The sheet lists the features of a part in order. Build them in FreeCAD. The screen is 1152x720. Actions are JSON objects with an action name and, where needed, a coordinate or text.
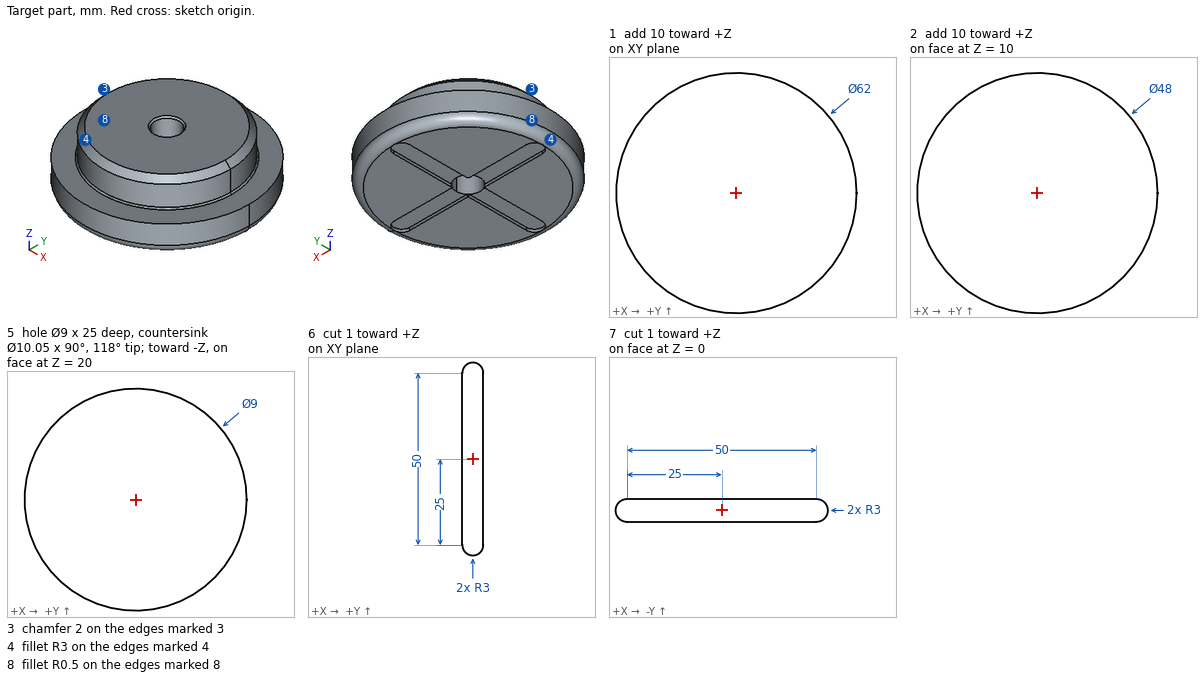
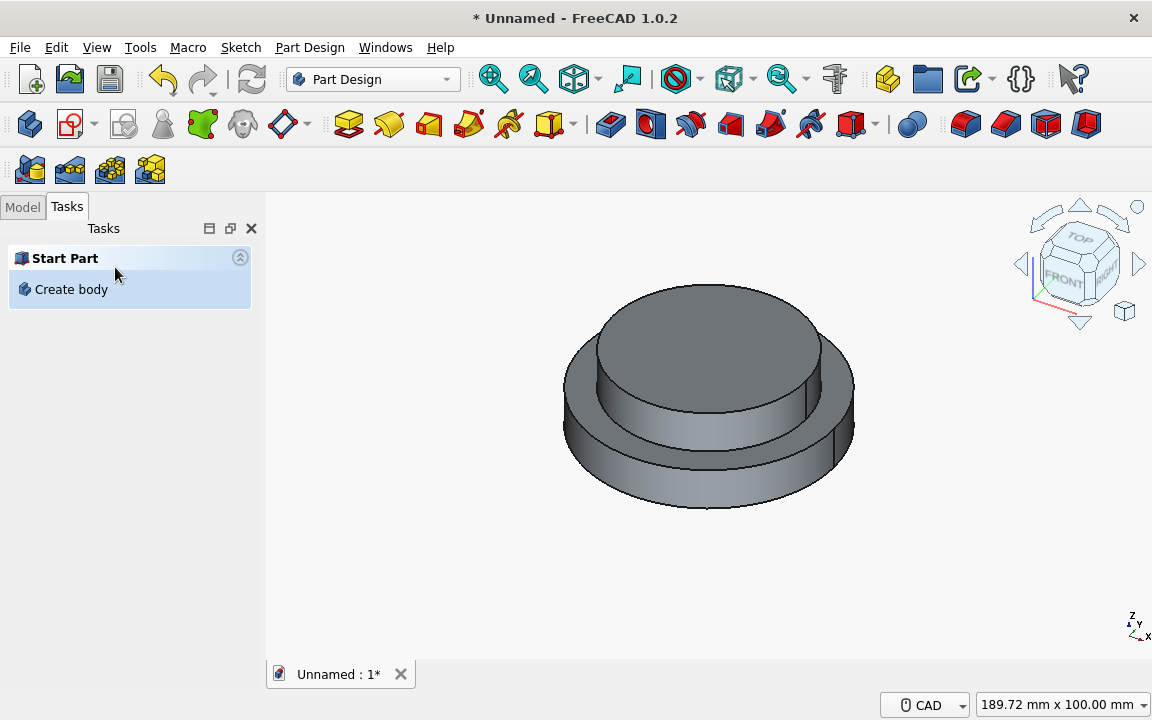
{"action": "left_click", "coordinate": [598, 355]}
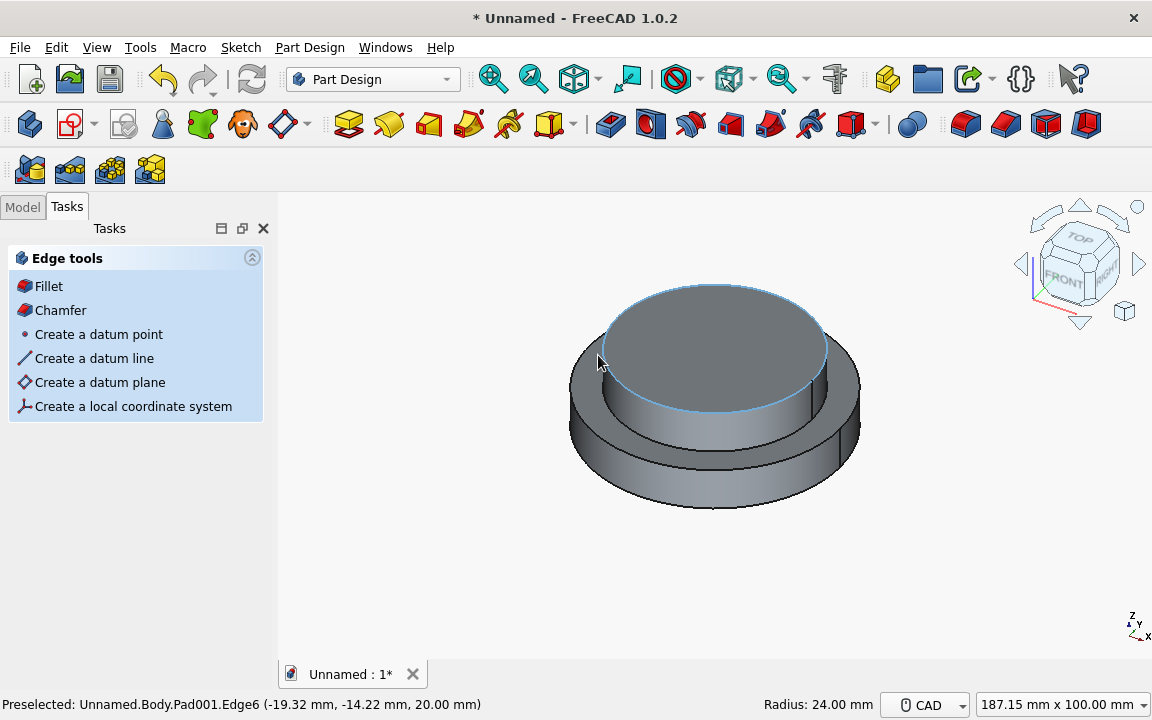
{"action": "left_click", "coordinate": [1006, 124]}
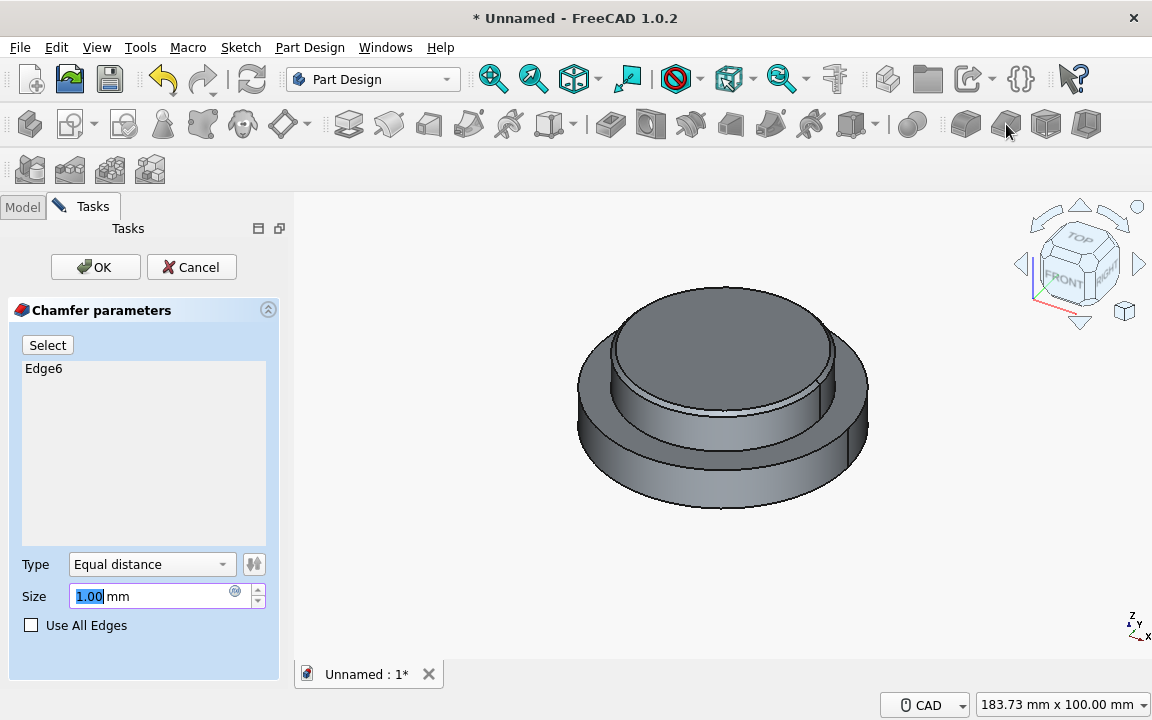
{"action": "type", "text": "2"}
{"action": "key", "text": "Tab"}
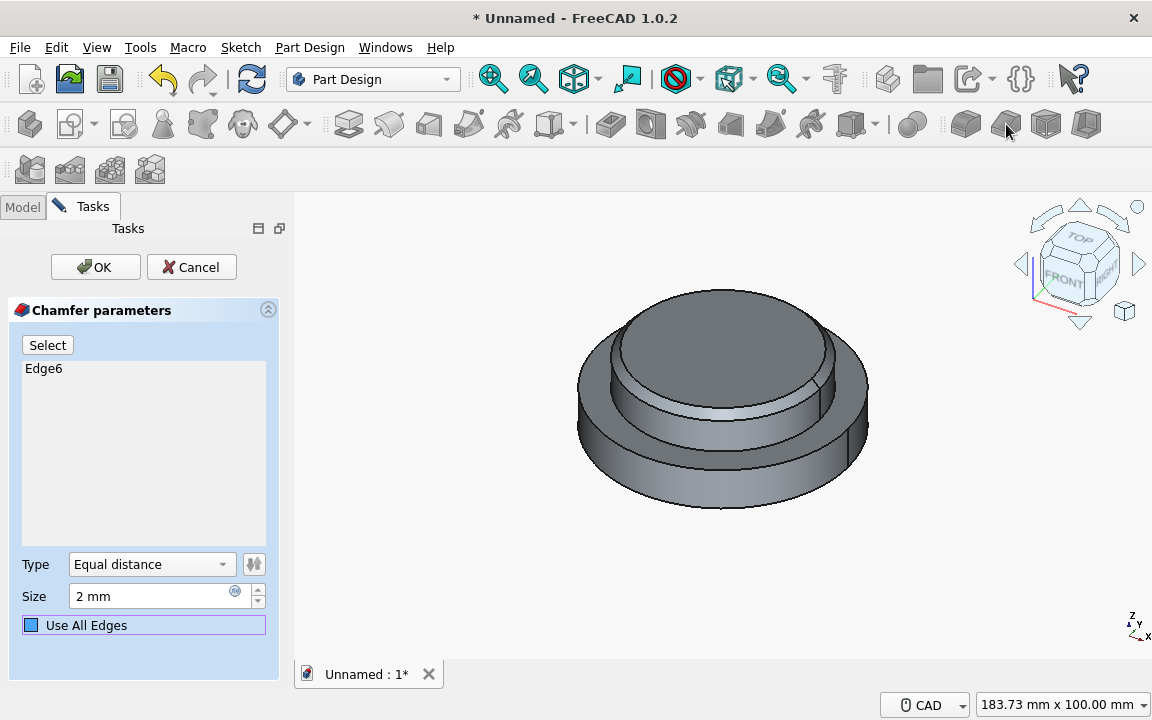
{"action": "left_click", "coordinate": [96, 267]}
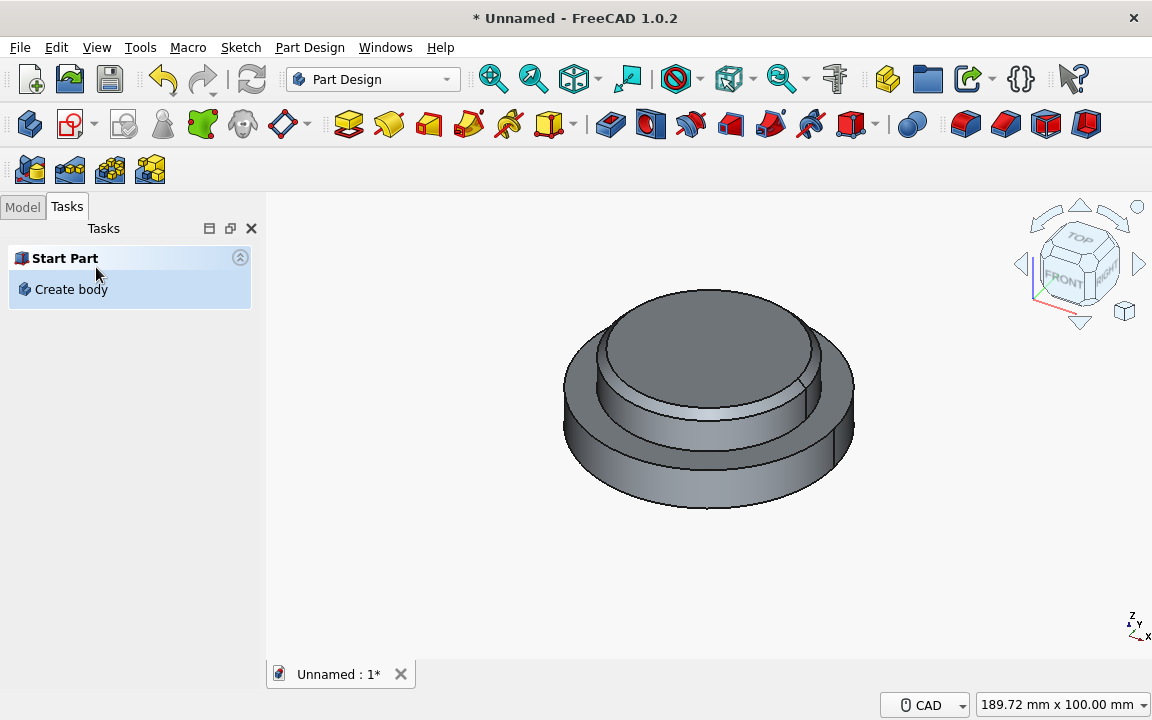
{"action": "key", "text": "0"}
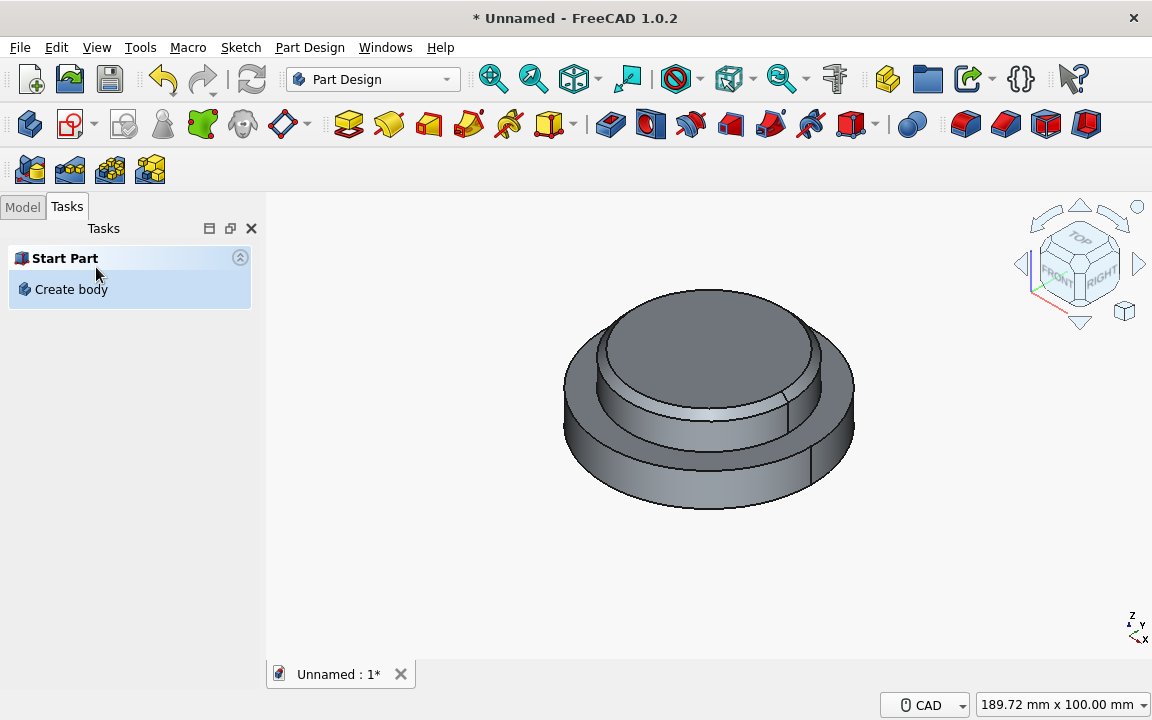
{"action": "key", "text": "2"}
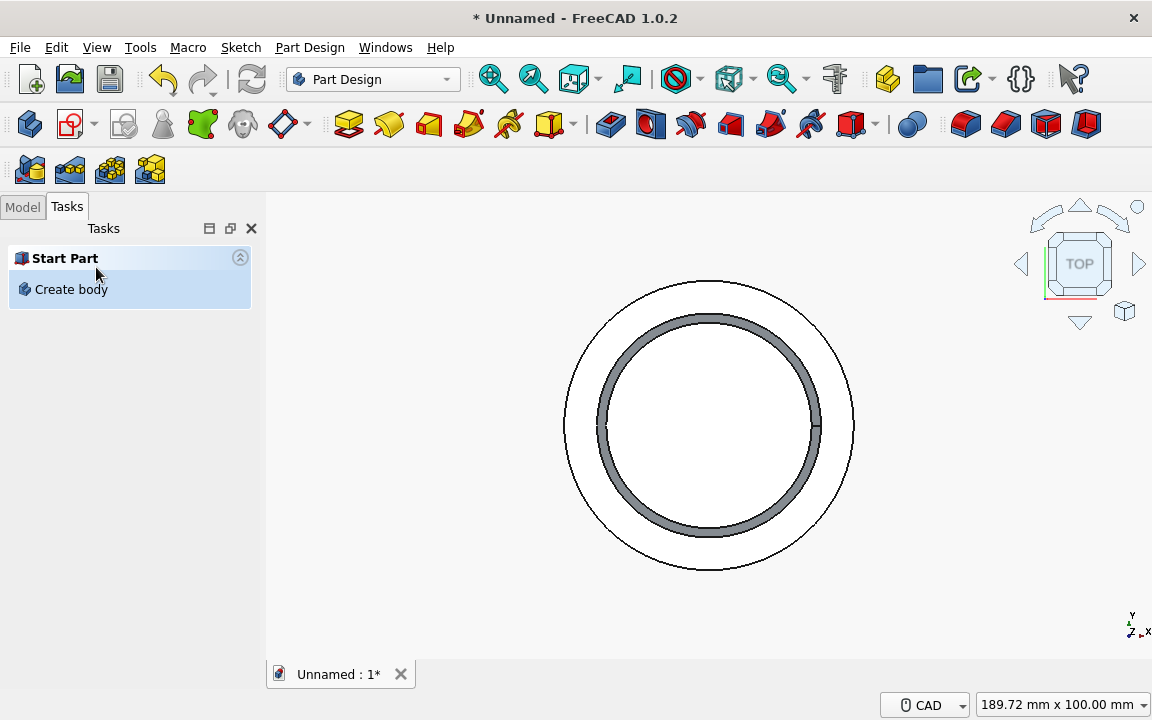
{"action": "key", "text": "1"}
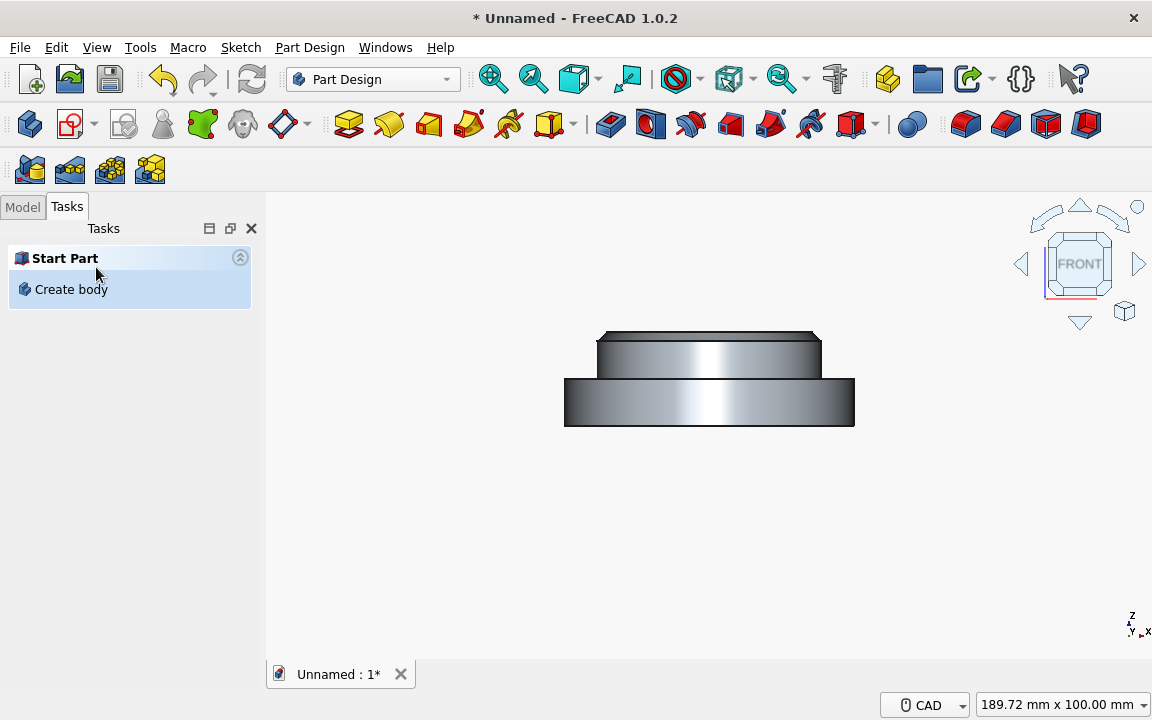
{"action": "left_click", "coordinate": [494, 80]}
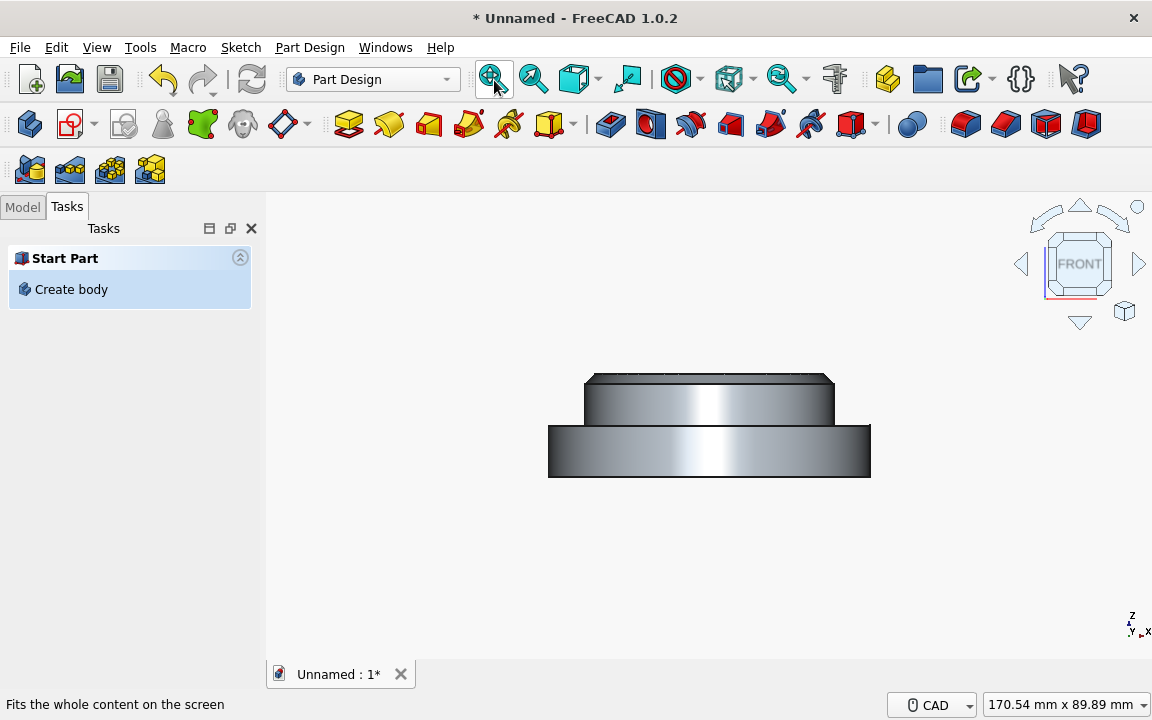
{"action": "left_click", "coordinate": [579, 476]}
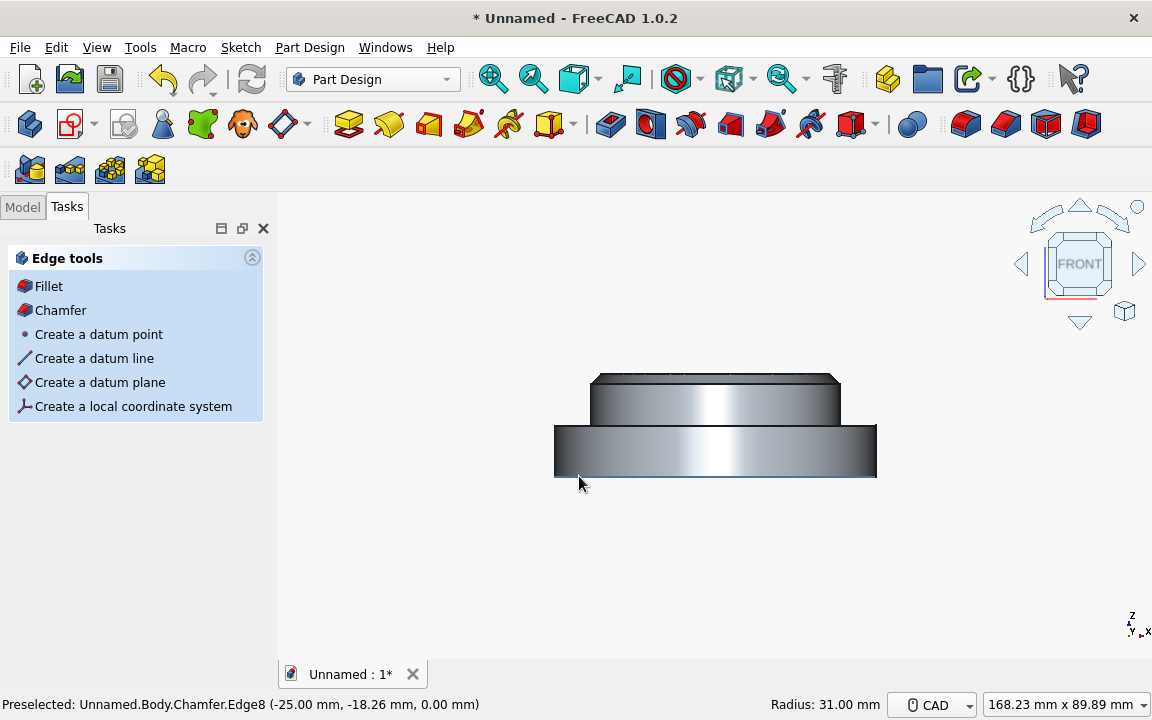
{"action": "left_click", "coordinate": [966, 124]}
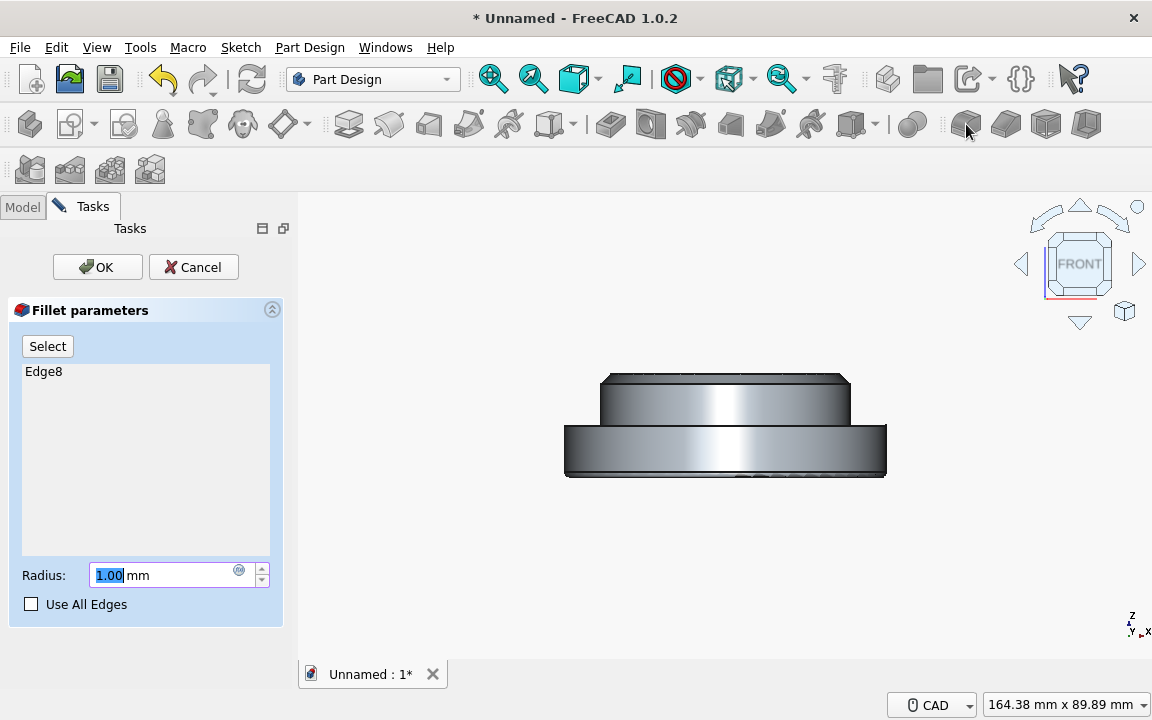
{"action": "type", "text": "3"}
{"action": "key", "text": "Tab"}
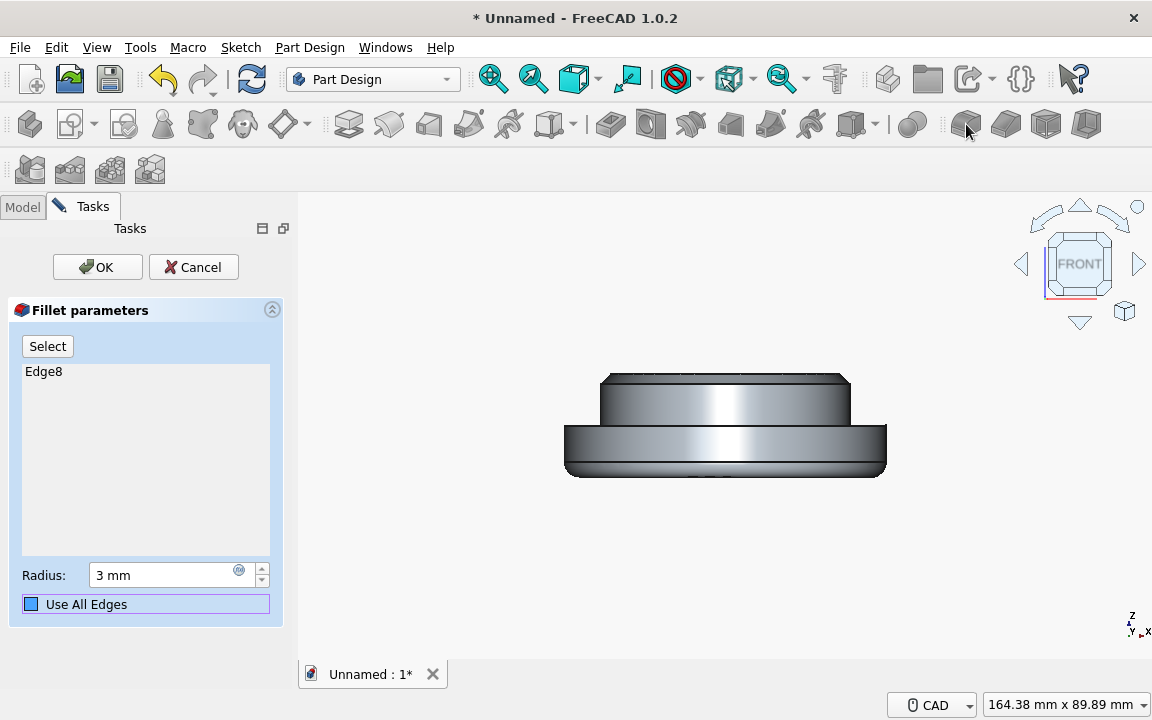
{"action": "left_click", "coordinate": [98, 267]}